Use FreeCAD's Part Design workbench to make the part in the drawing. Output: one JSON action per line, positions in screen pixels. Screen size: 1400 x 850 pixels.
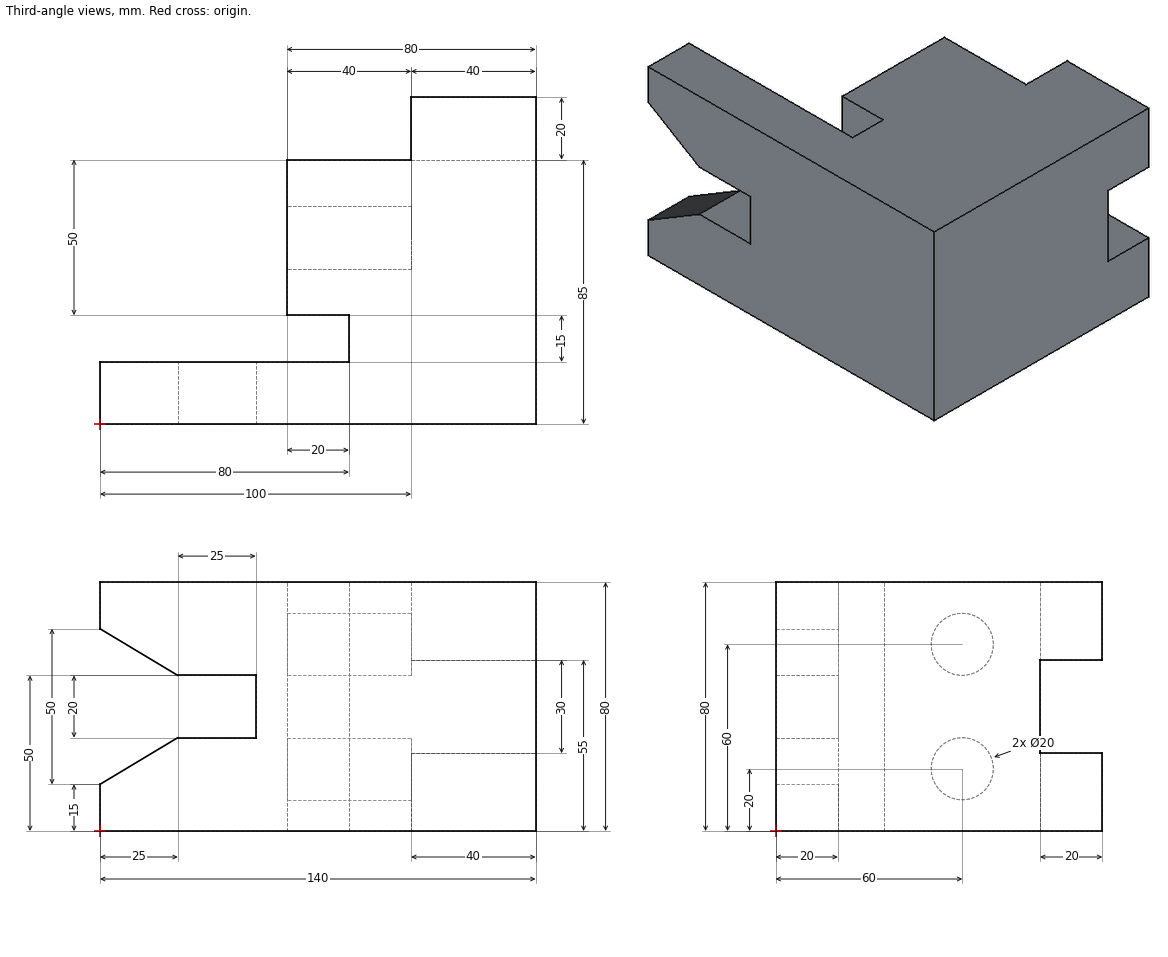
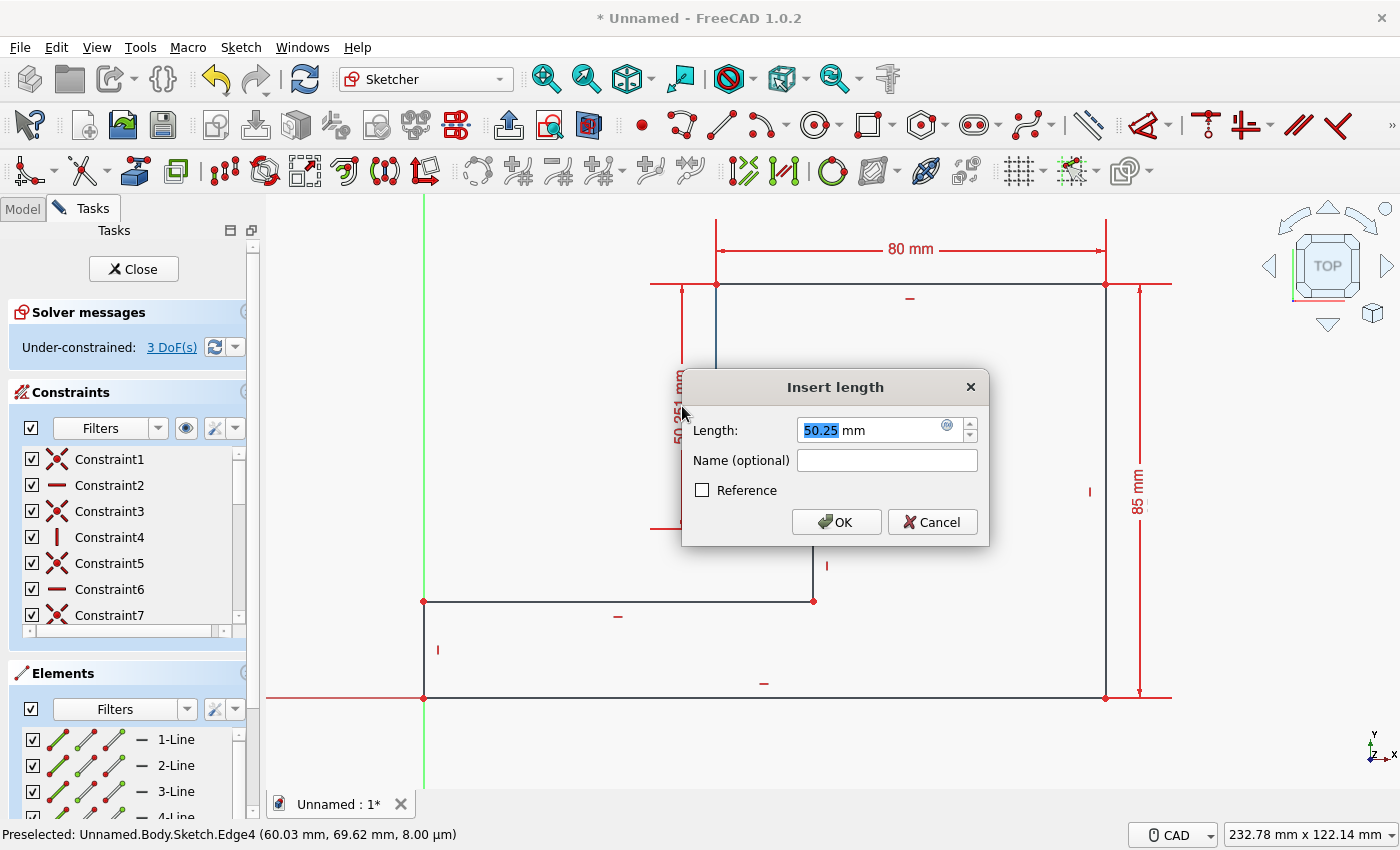
{"action": "type", "text": "50"}
{"action": "key", "text": "Return"}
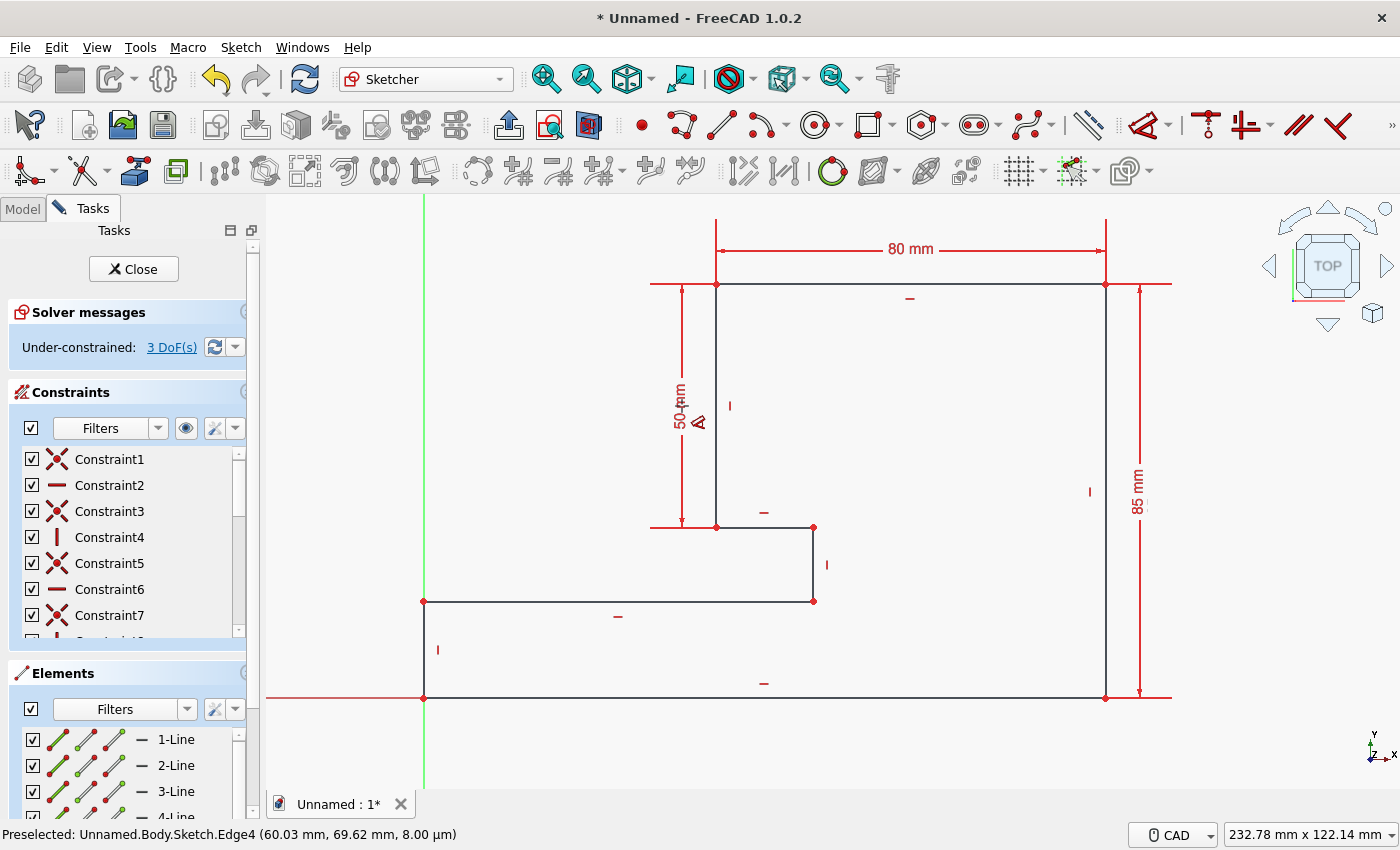
{"action": "left_click", "coordinate": [745, 528]}
{"action": "left_click", "coordinate": [765, 562]}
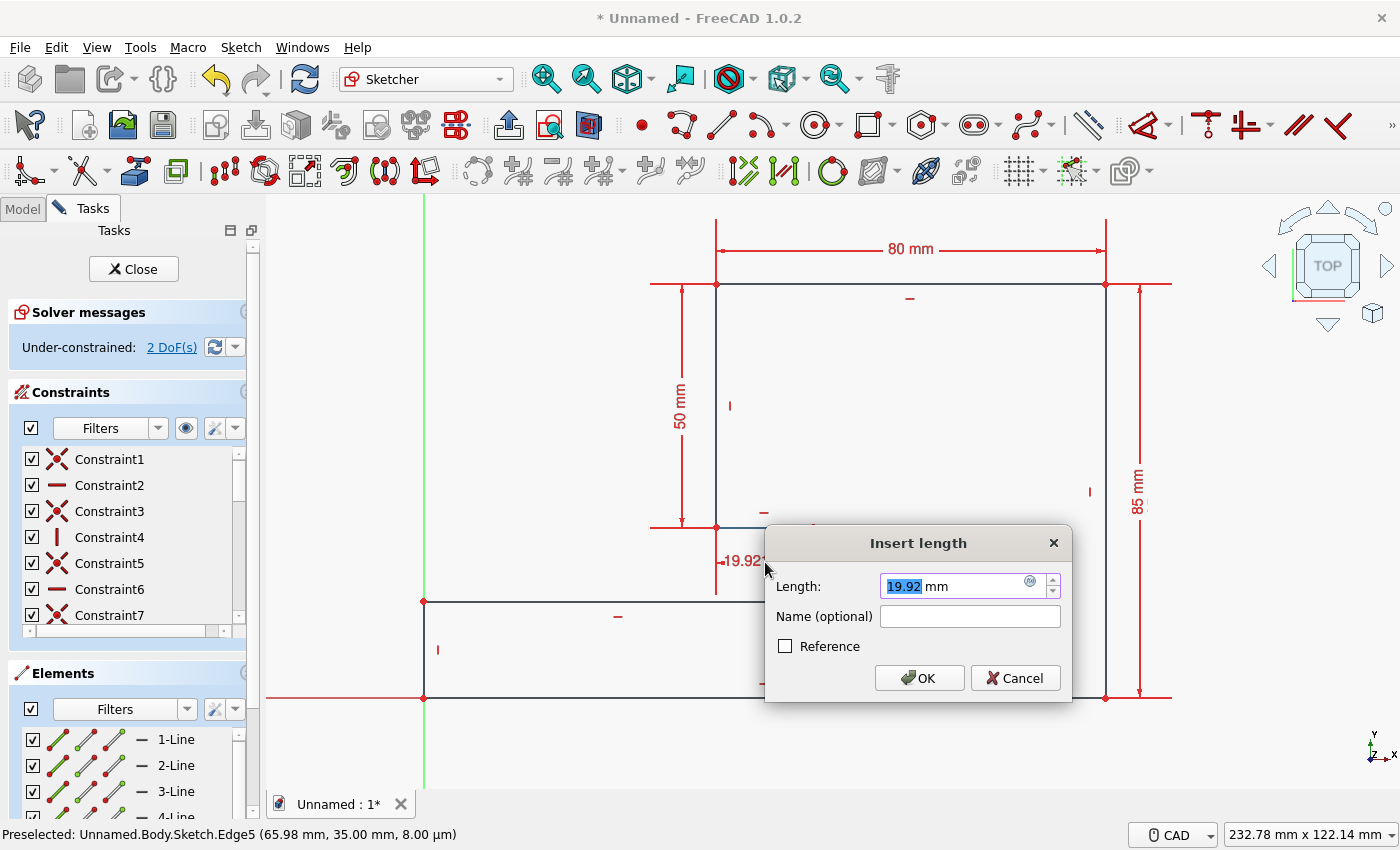
{"action": "type", "text": "20"}
{"action": "key", "text": "Return"}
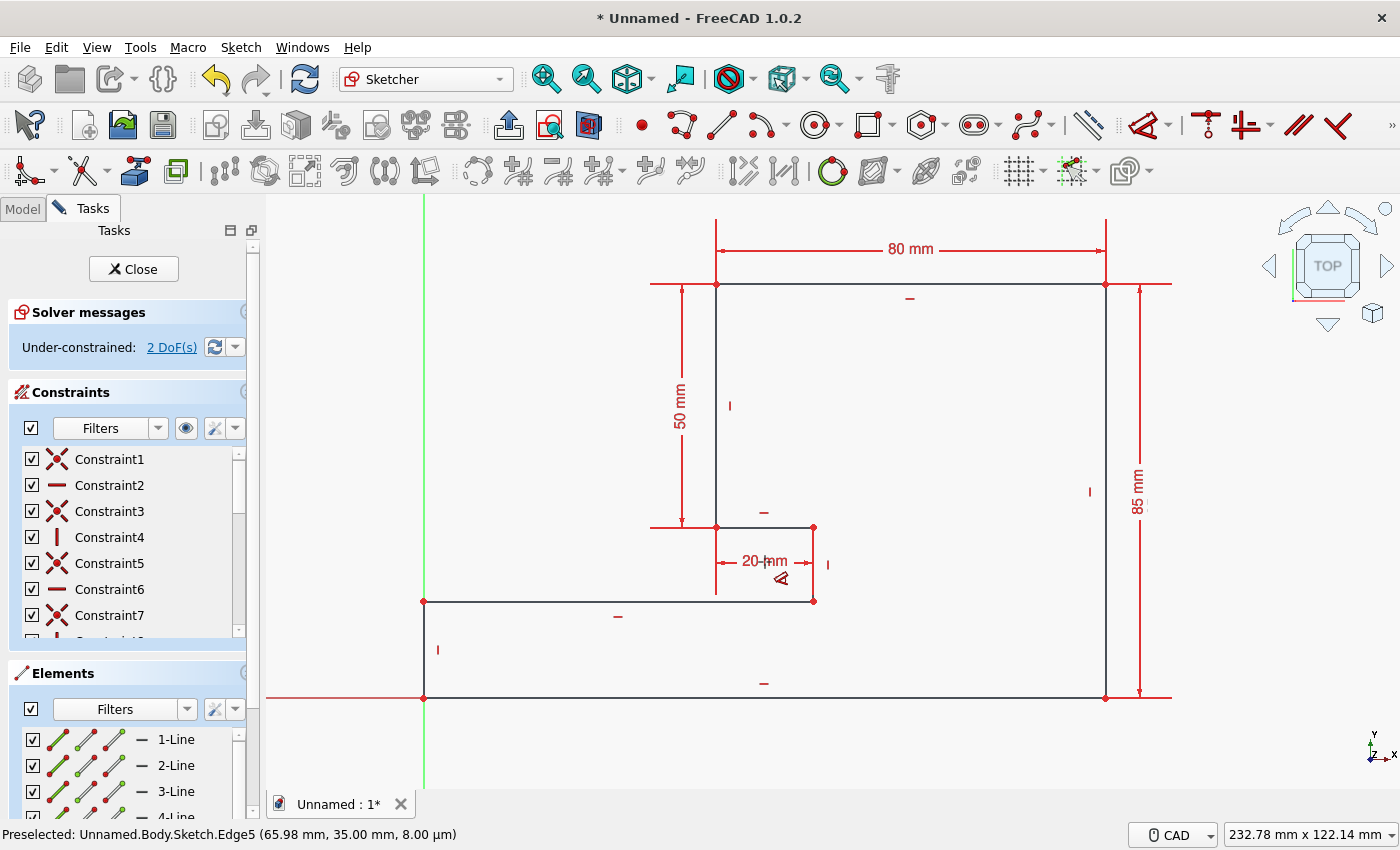
{"action": "left_click", "coordinate": [813, 550]}
{"action": "left_click", "coordinate": [847, 565]}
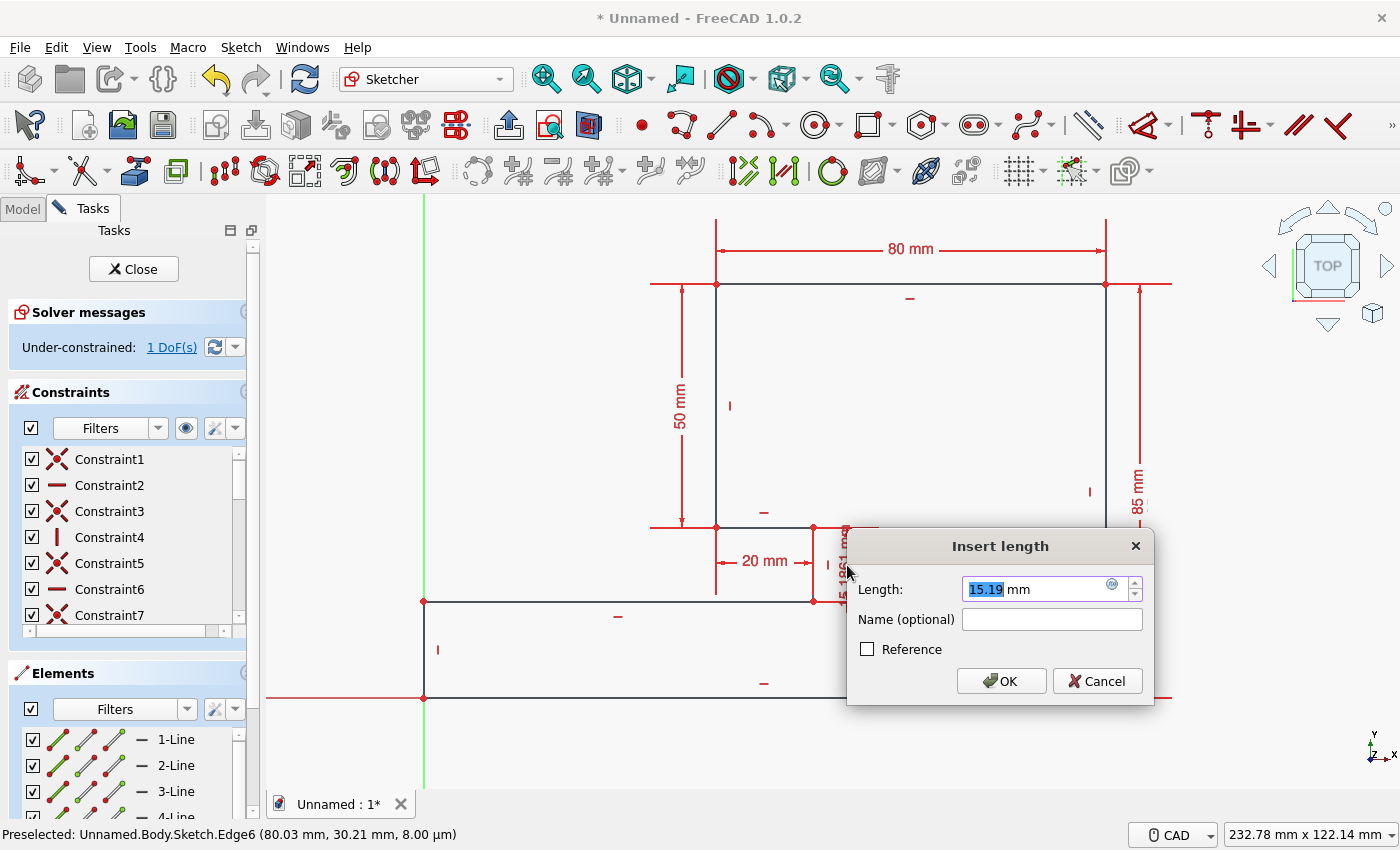
{"action": "type", "text": "15"}
{"action": "key", "text": "Return"}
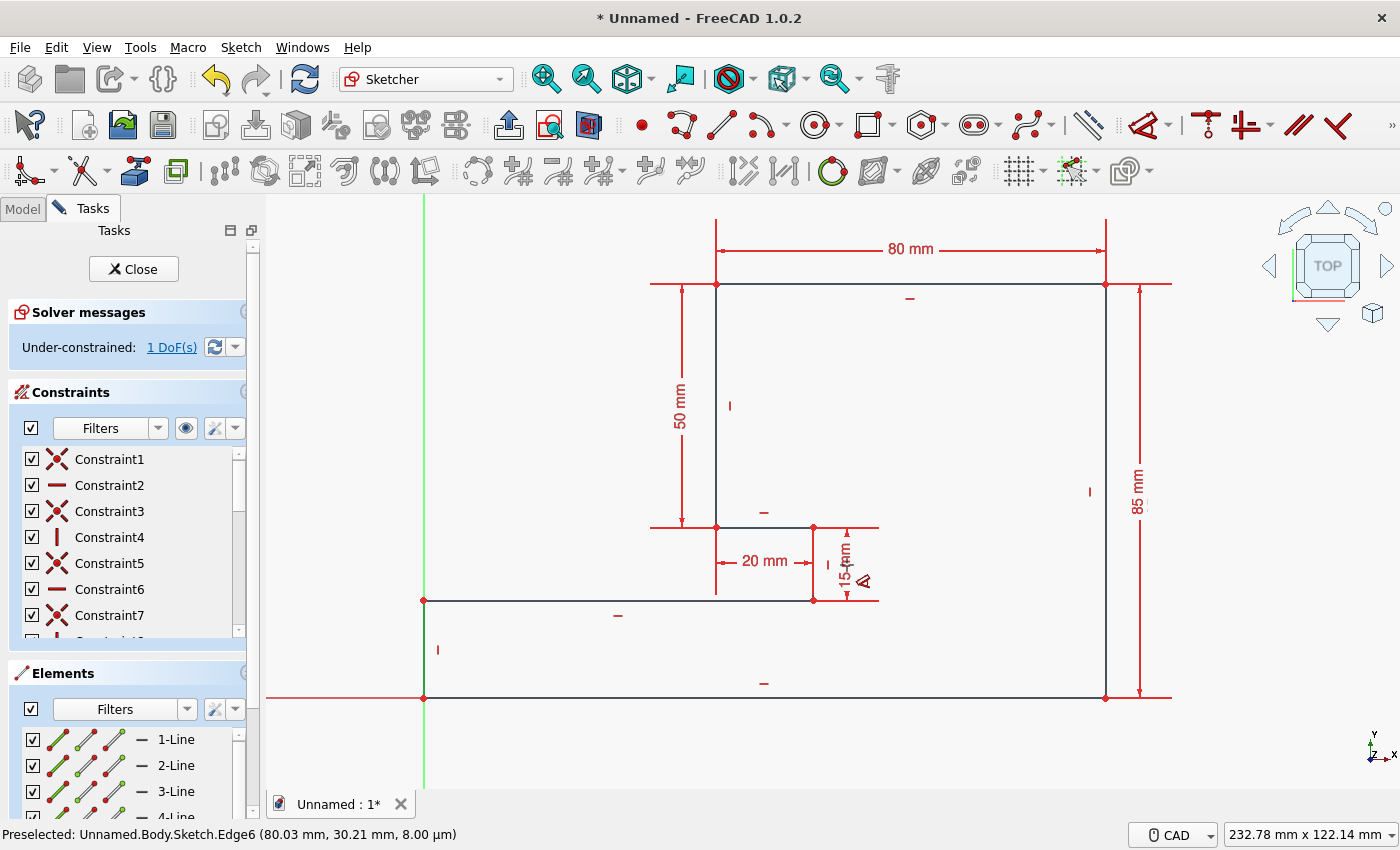
{"action": "left_click", "coordinate": [696, 601]}
{"action": "left_click", "coordinate": [619, 635]}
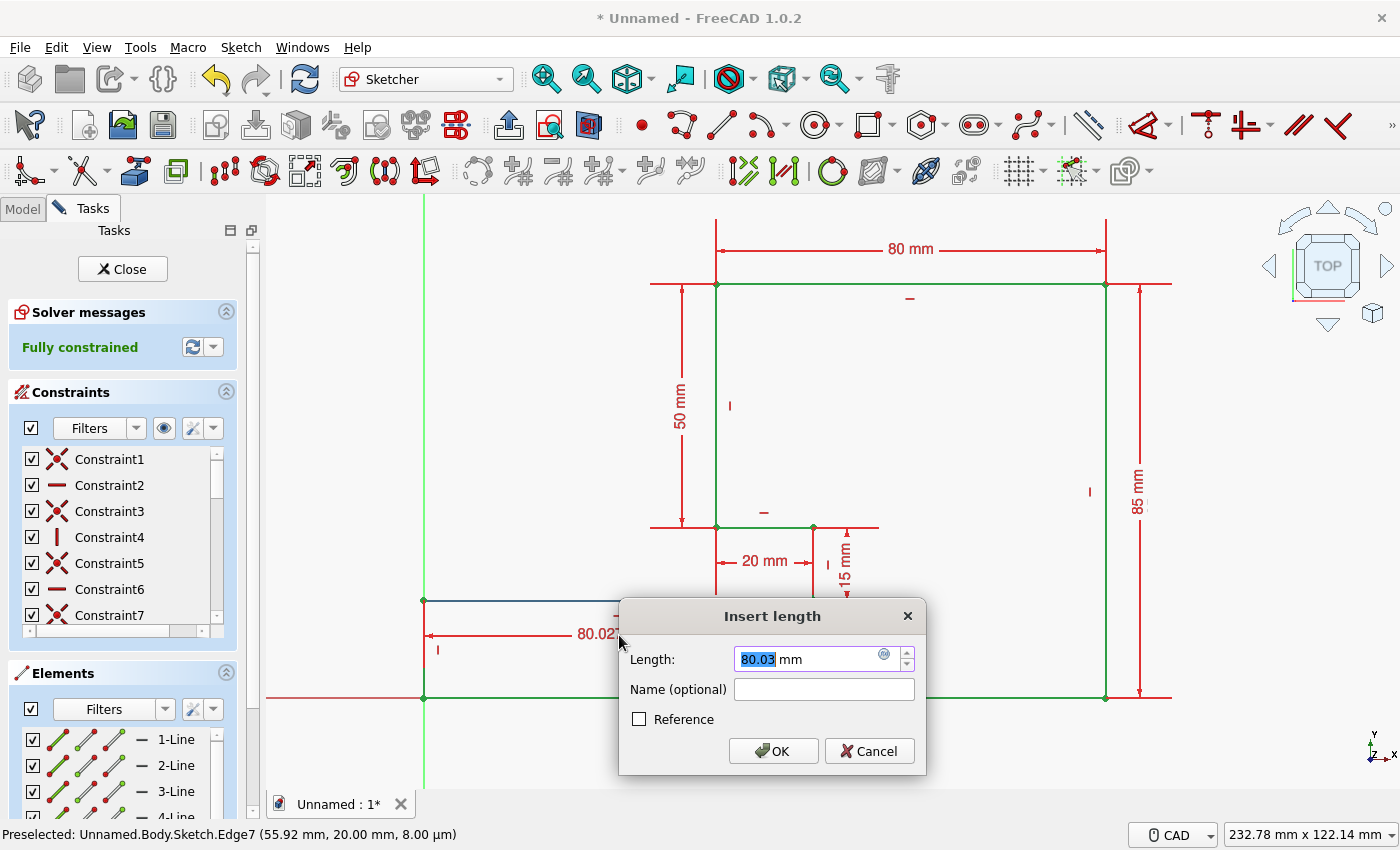
{"action": "type", "text": "80"}
{"action": "key", "text": "Return"}
{"action": "key", "text": "Escape"}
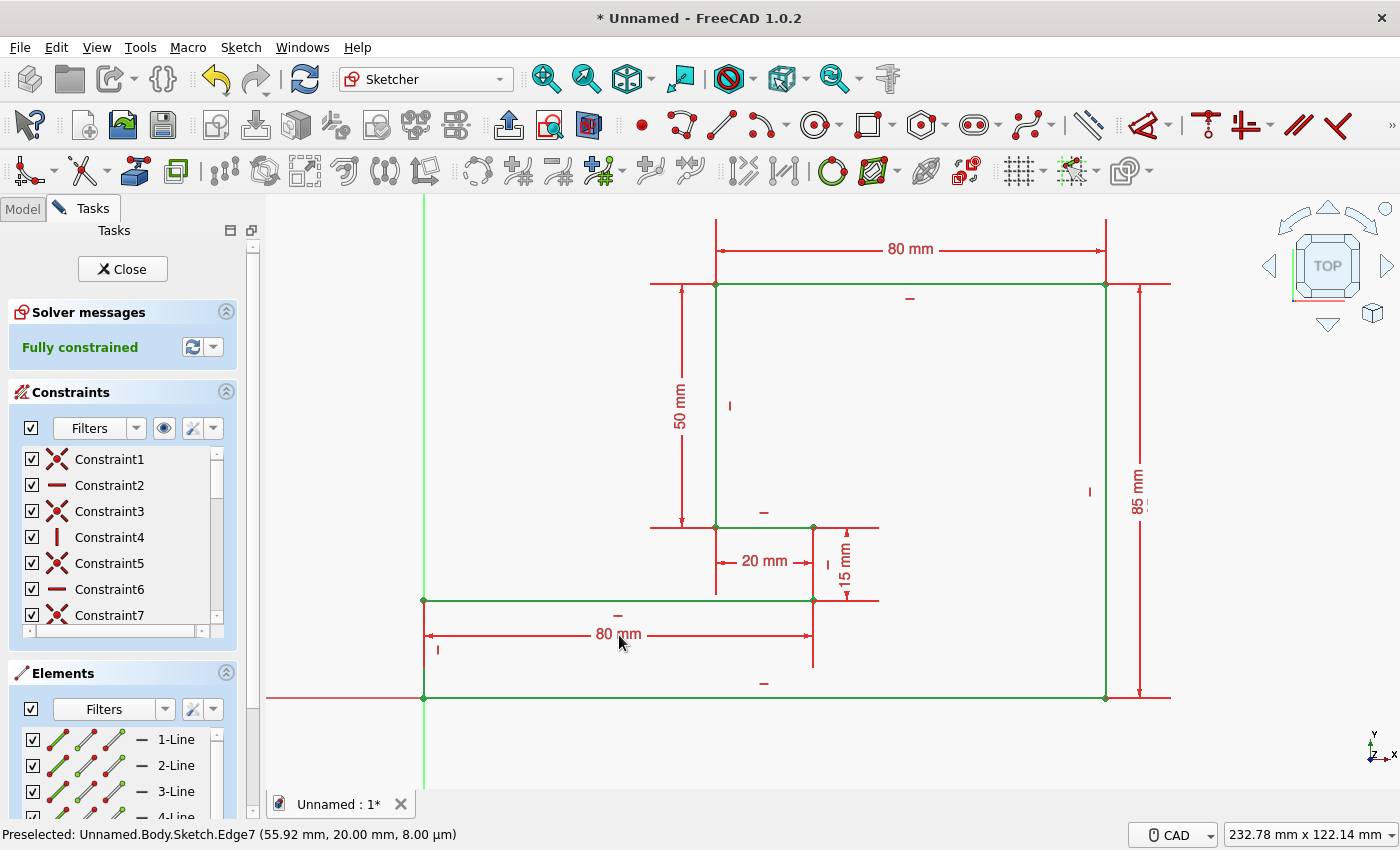
{"action": "left_click", "coordinate": [123, 269]}